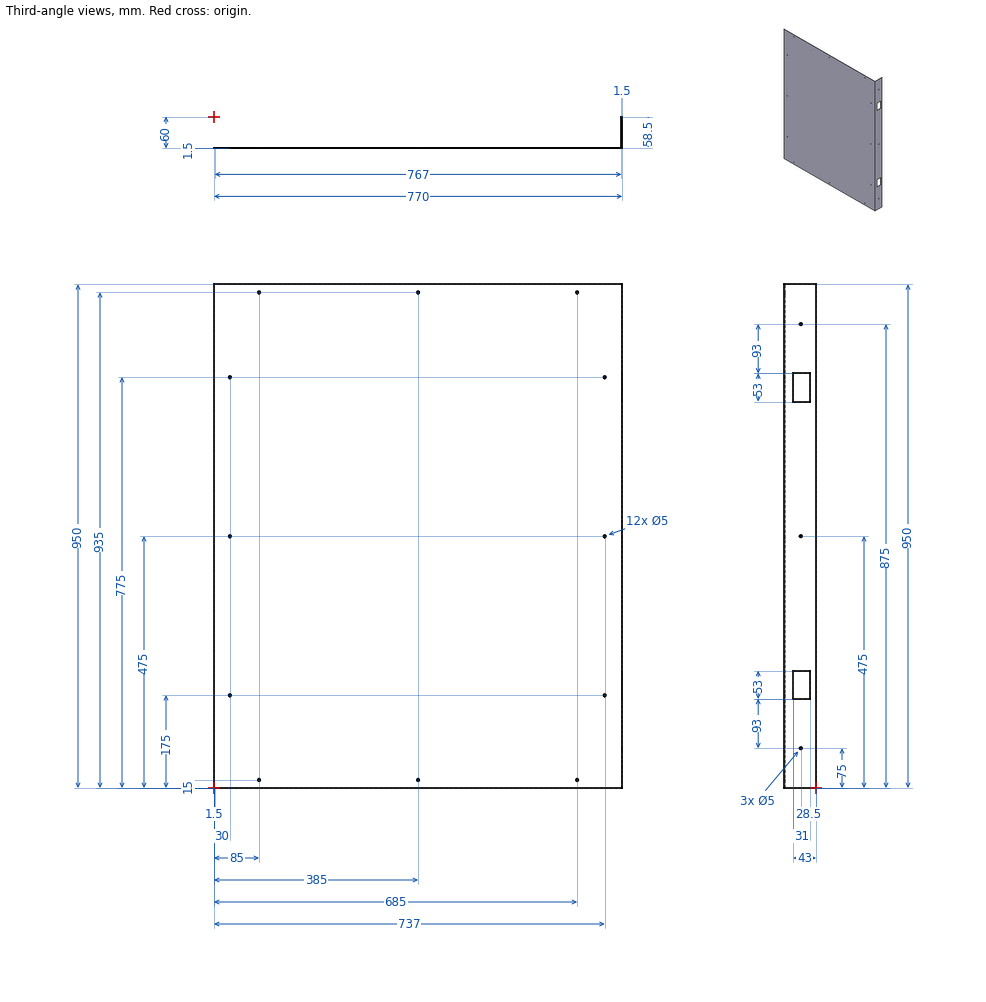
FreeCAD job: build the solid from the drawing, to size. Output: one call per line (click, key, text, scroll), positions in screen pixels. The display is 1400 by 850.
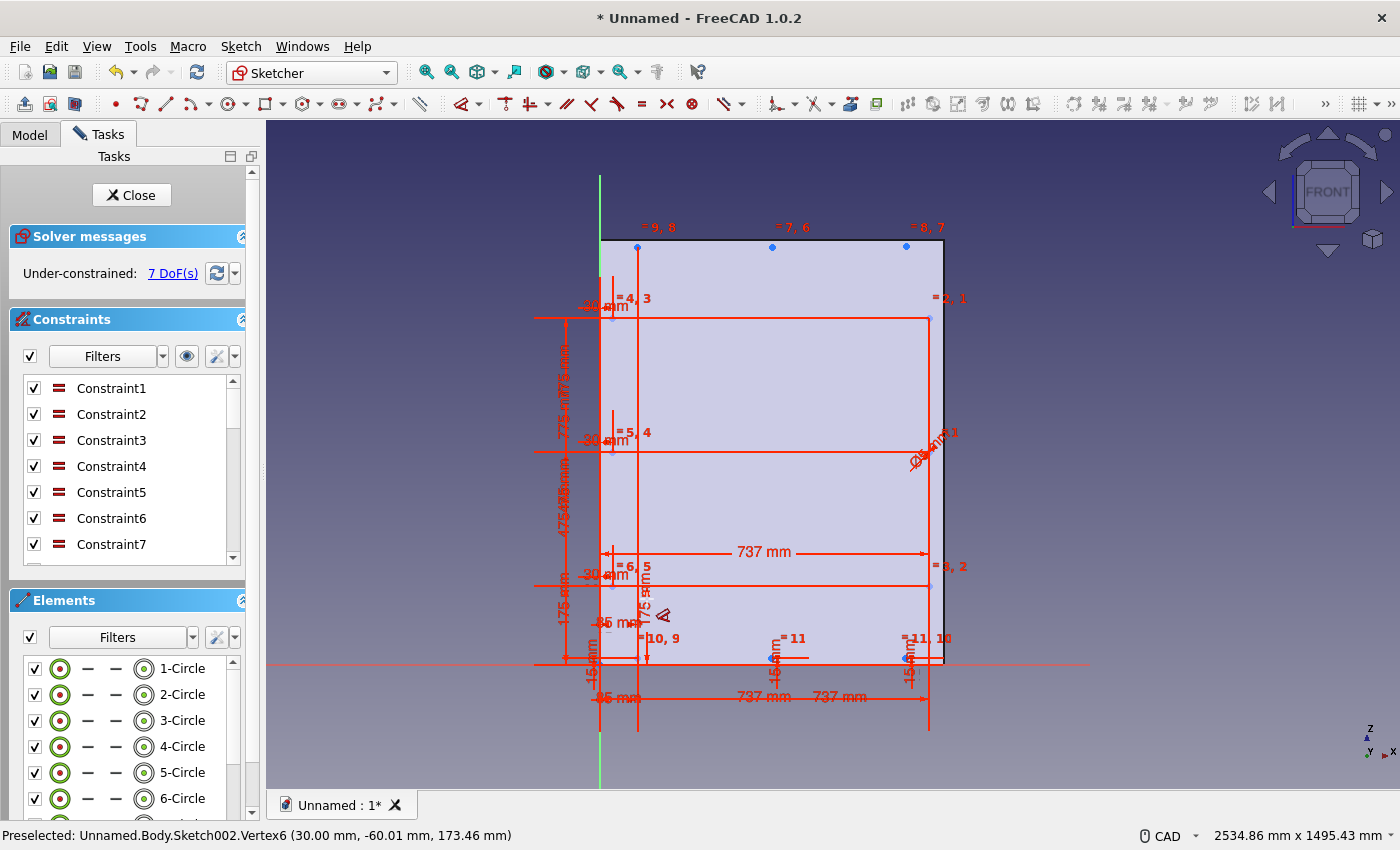
click(772, 247)
click(686, 213)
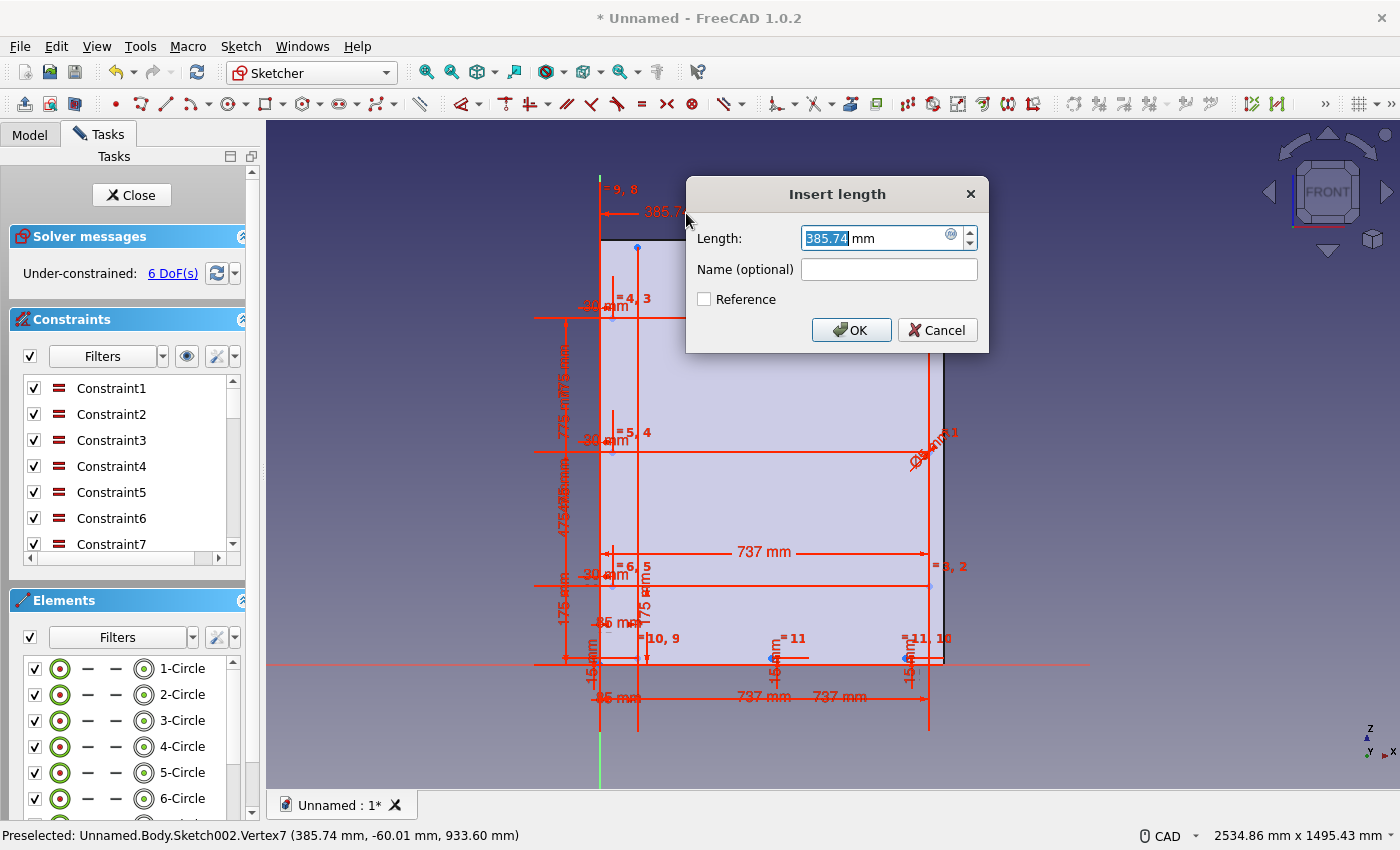
text(385)
key(Return)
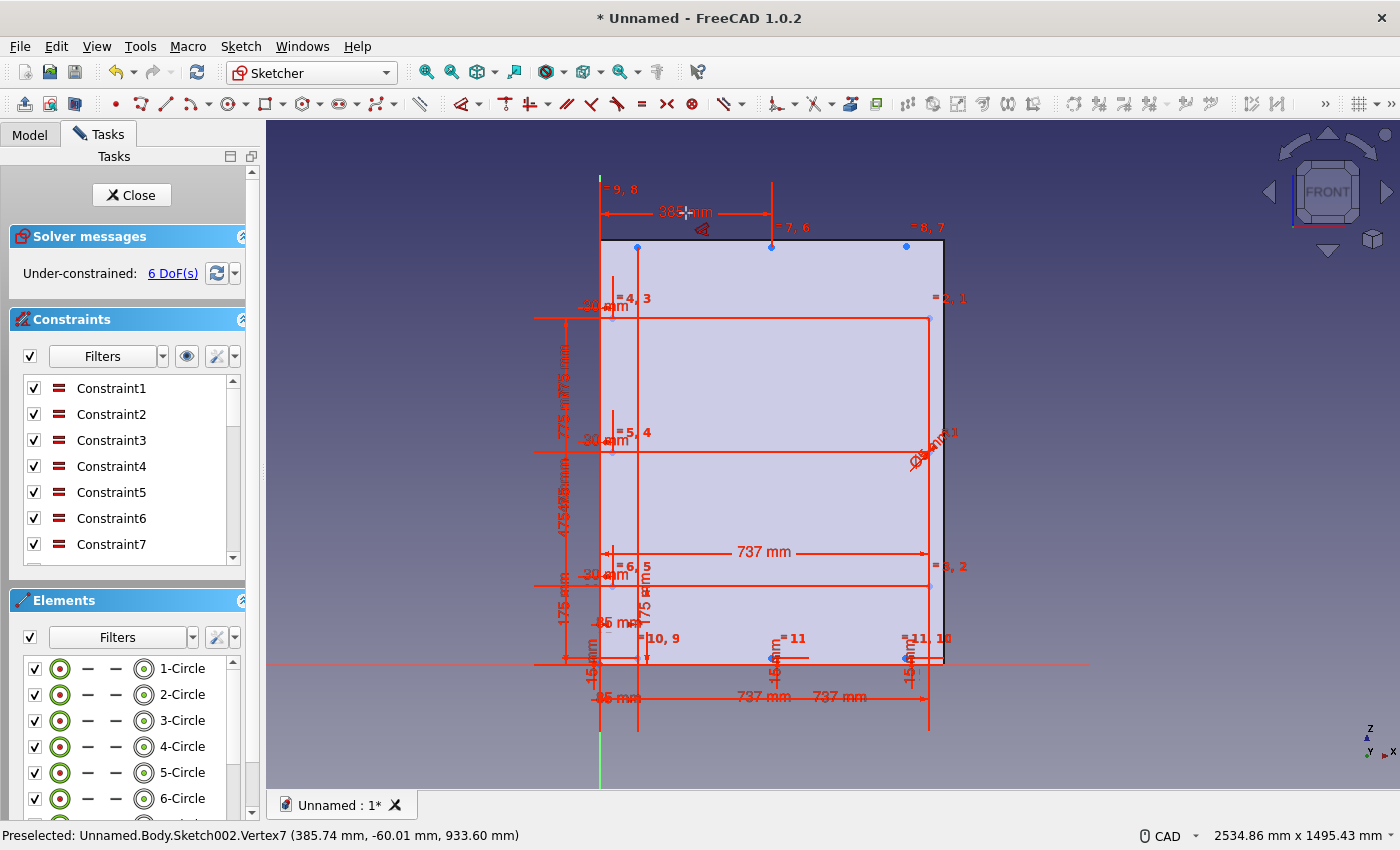
click(772, 247)
click(566, 552)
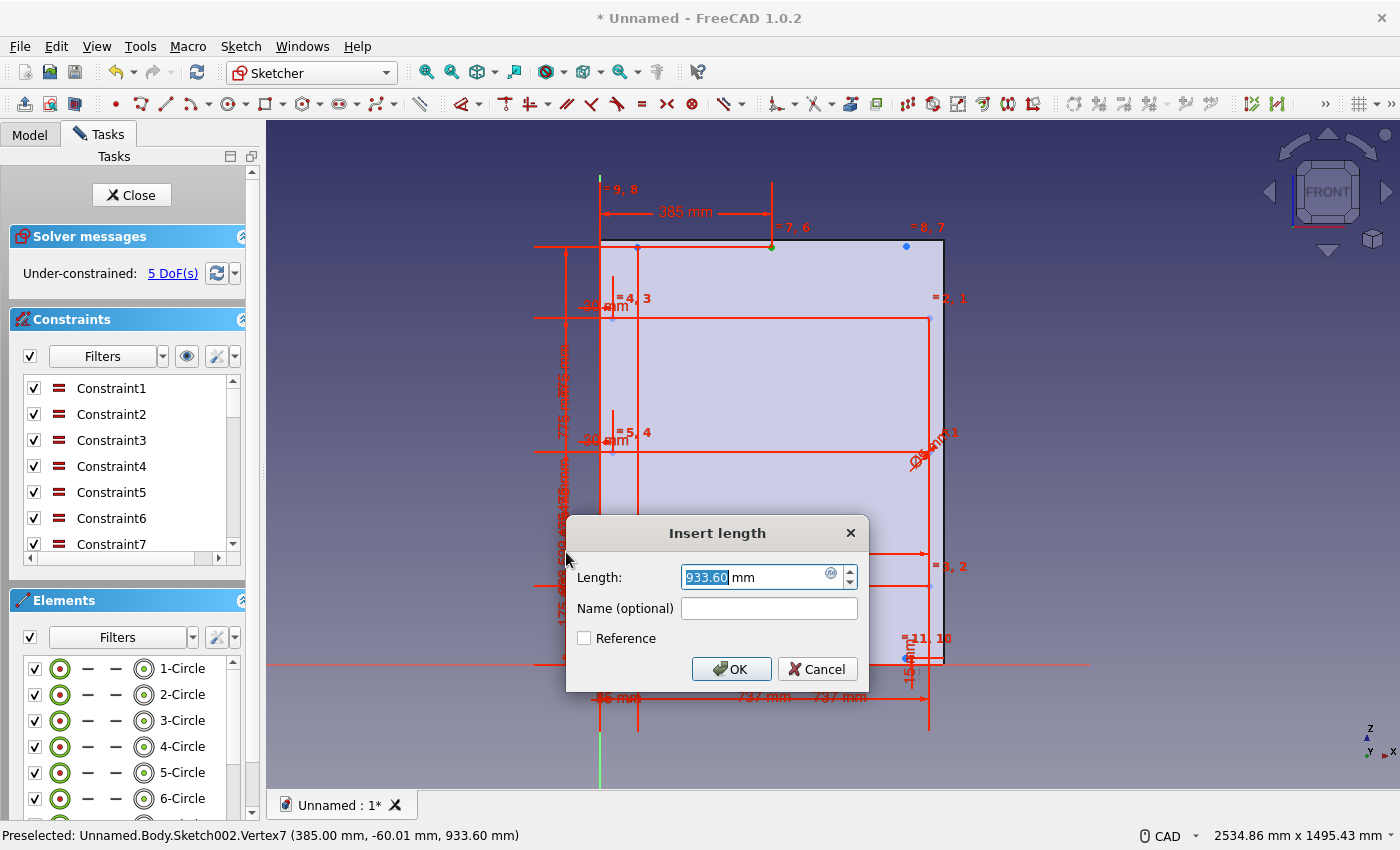
text(935)
key(Return)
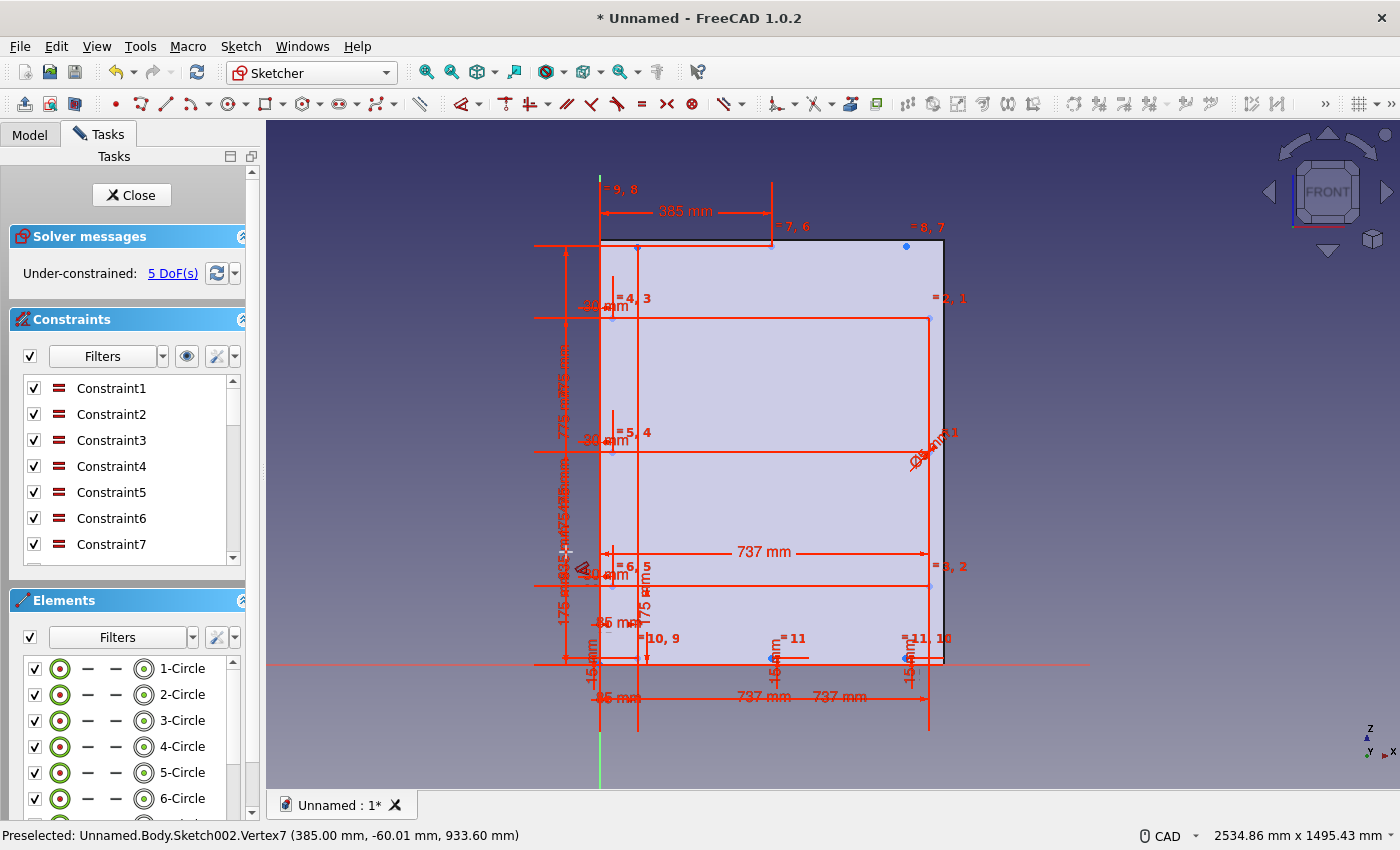
click(906, 247)
click(824, 213)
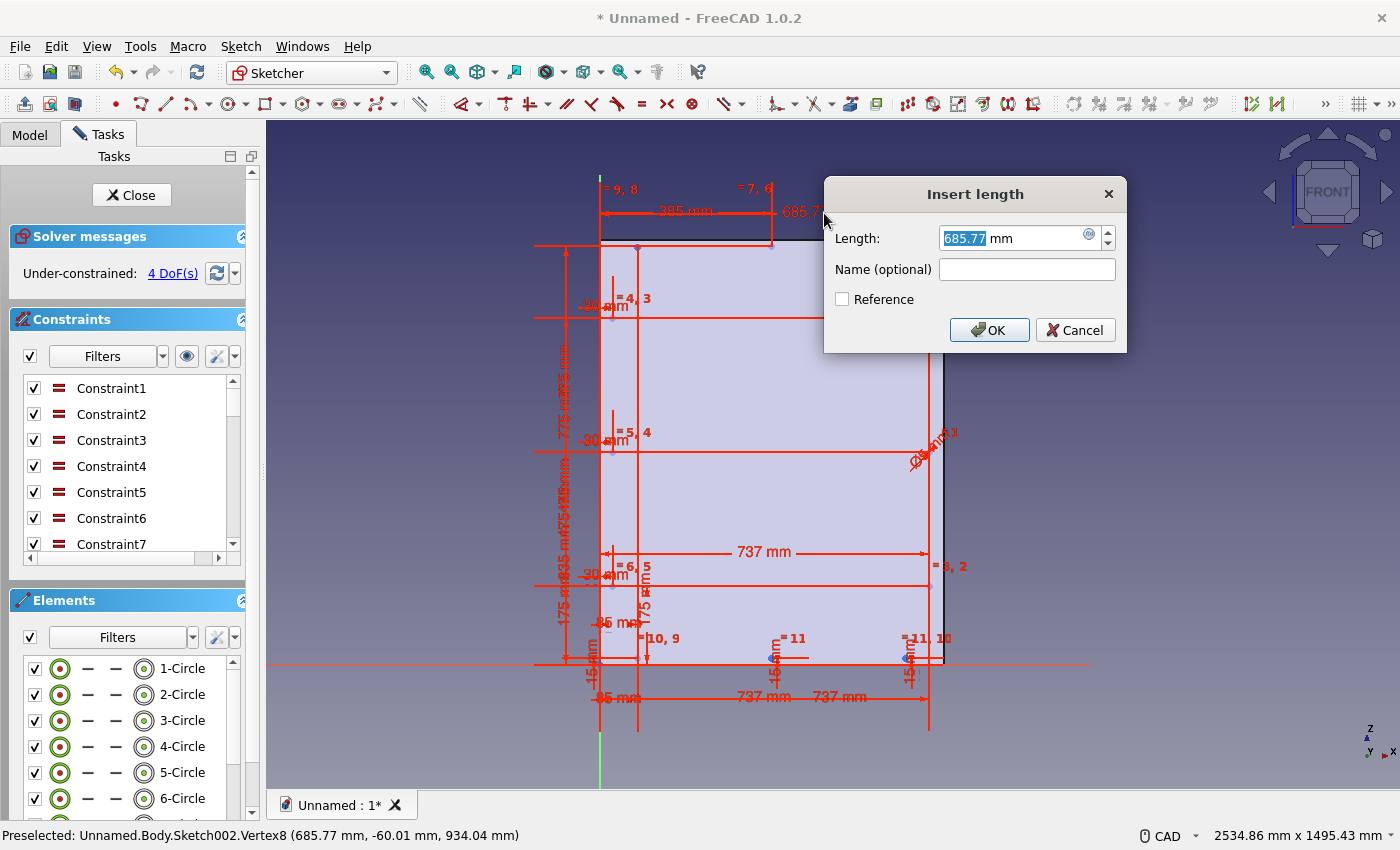
text(685)
key(Return)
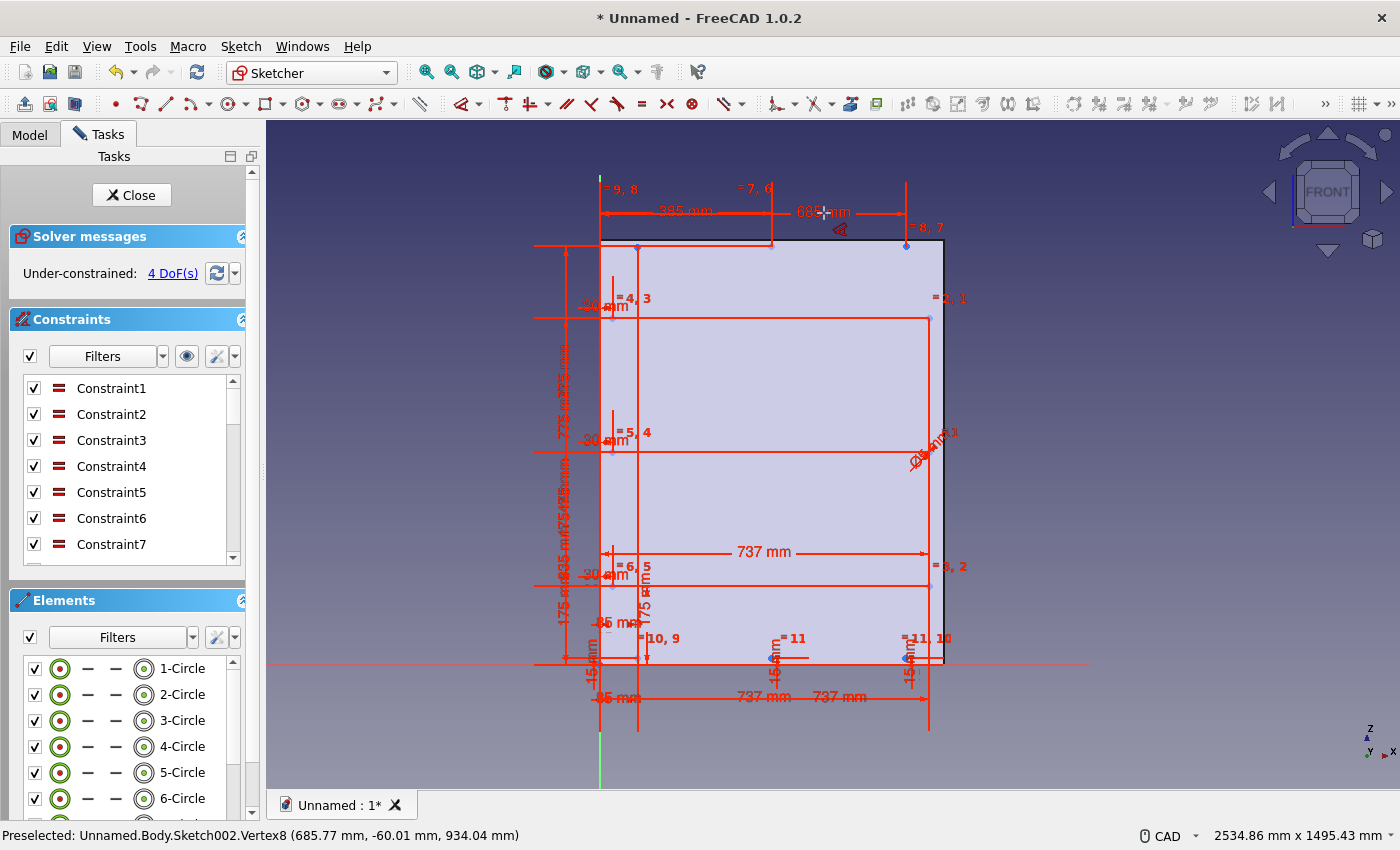
click(906, 247)
click(940, 360)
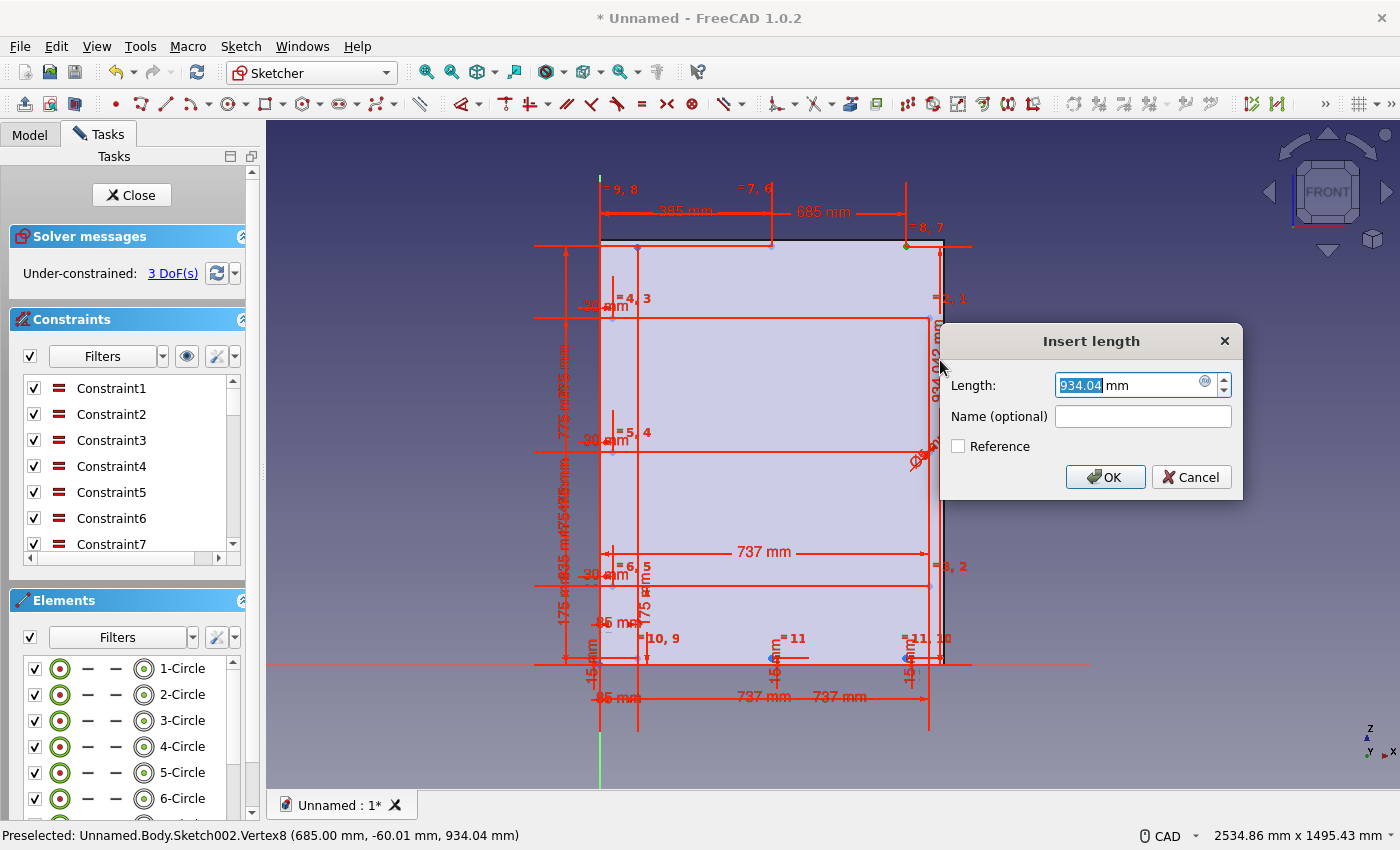
text(935)
key(Return)